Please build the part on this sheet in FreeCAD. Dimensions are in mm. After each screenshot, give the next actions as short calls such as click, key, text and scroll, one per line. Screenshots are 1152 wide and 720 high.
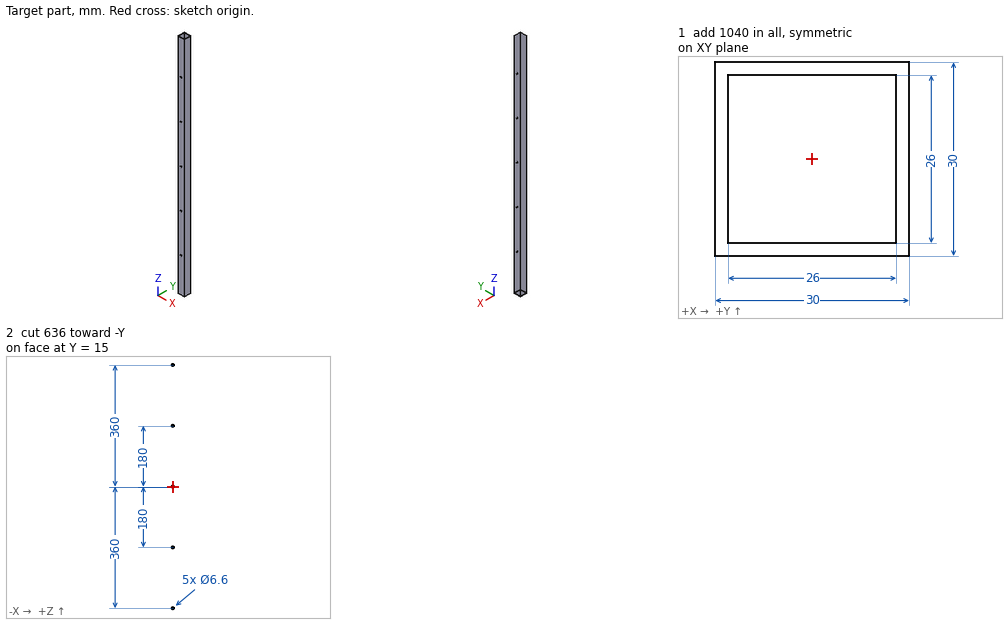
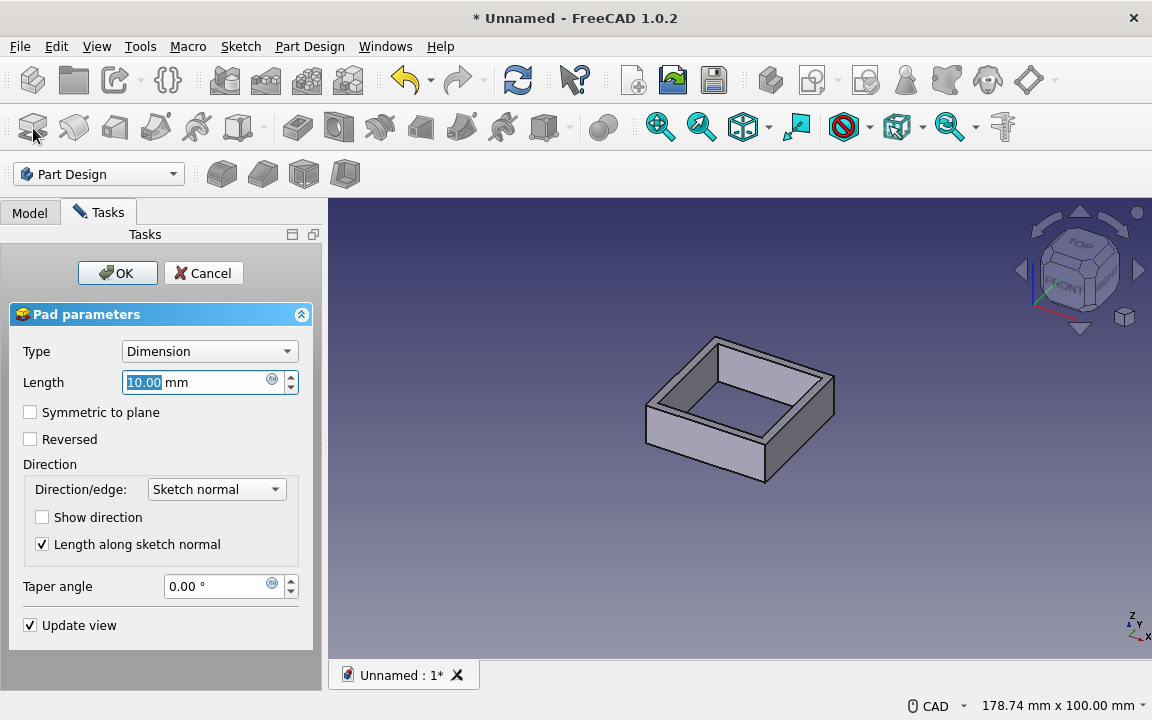
text(1040)
key(Tab)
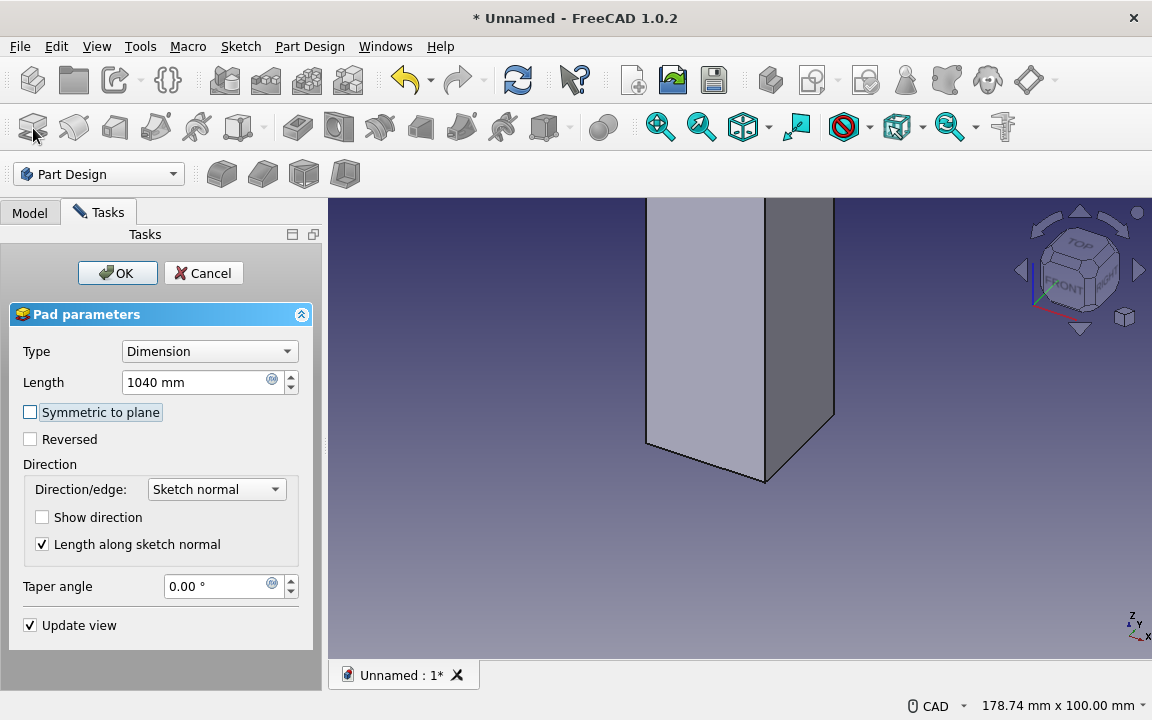
click(31, 412)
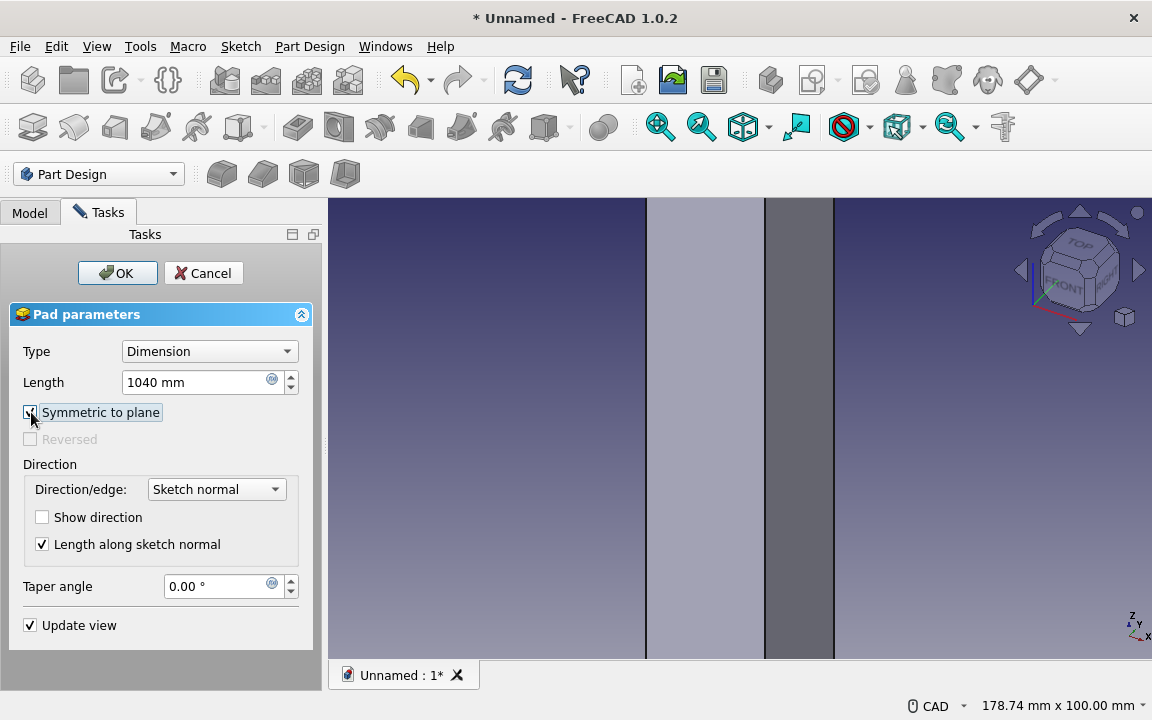
click(118, 273)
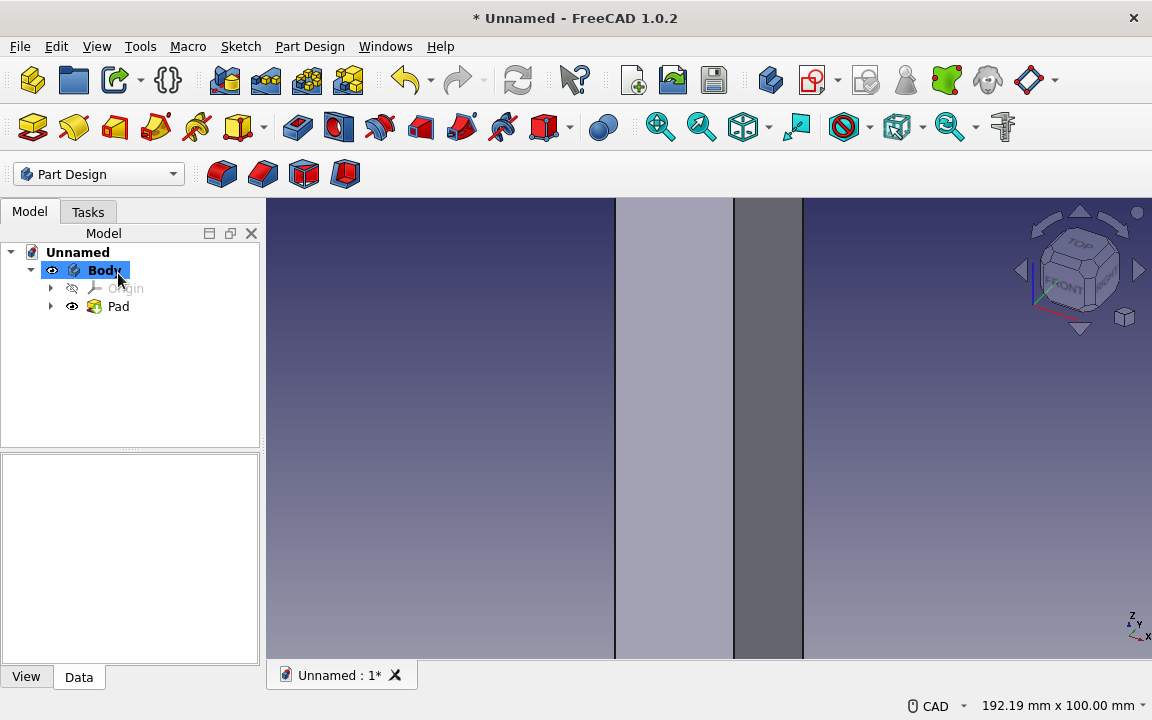
key(v)
key(f)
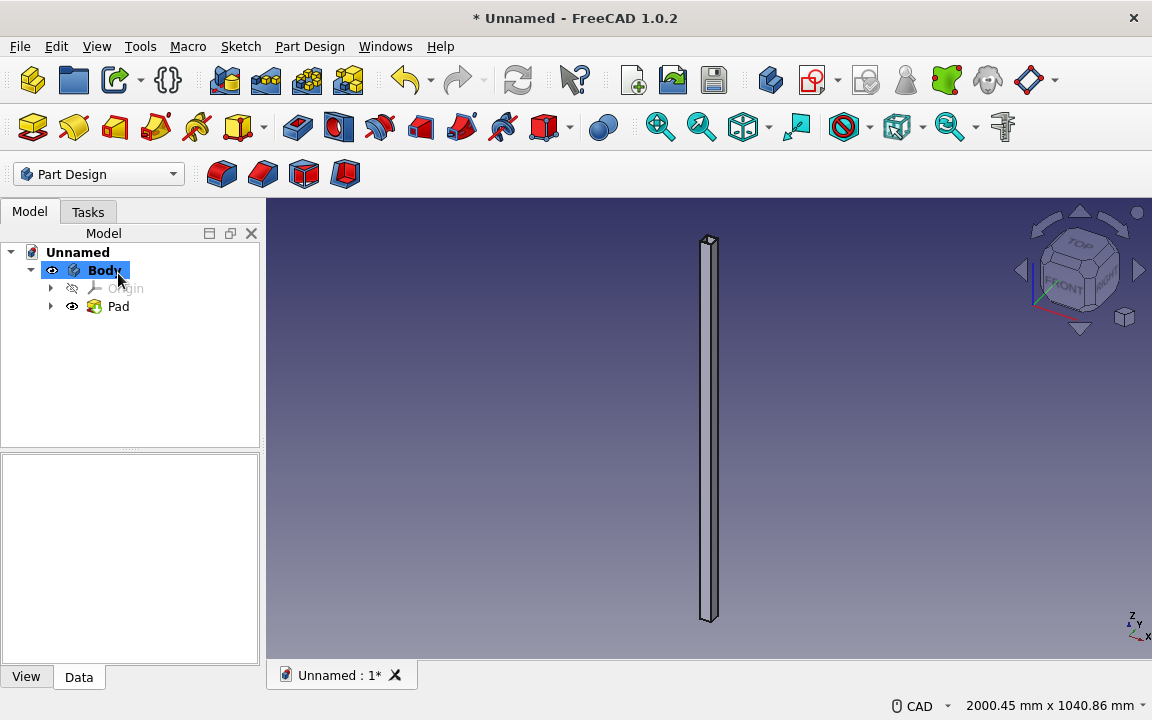
key(4)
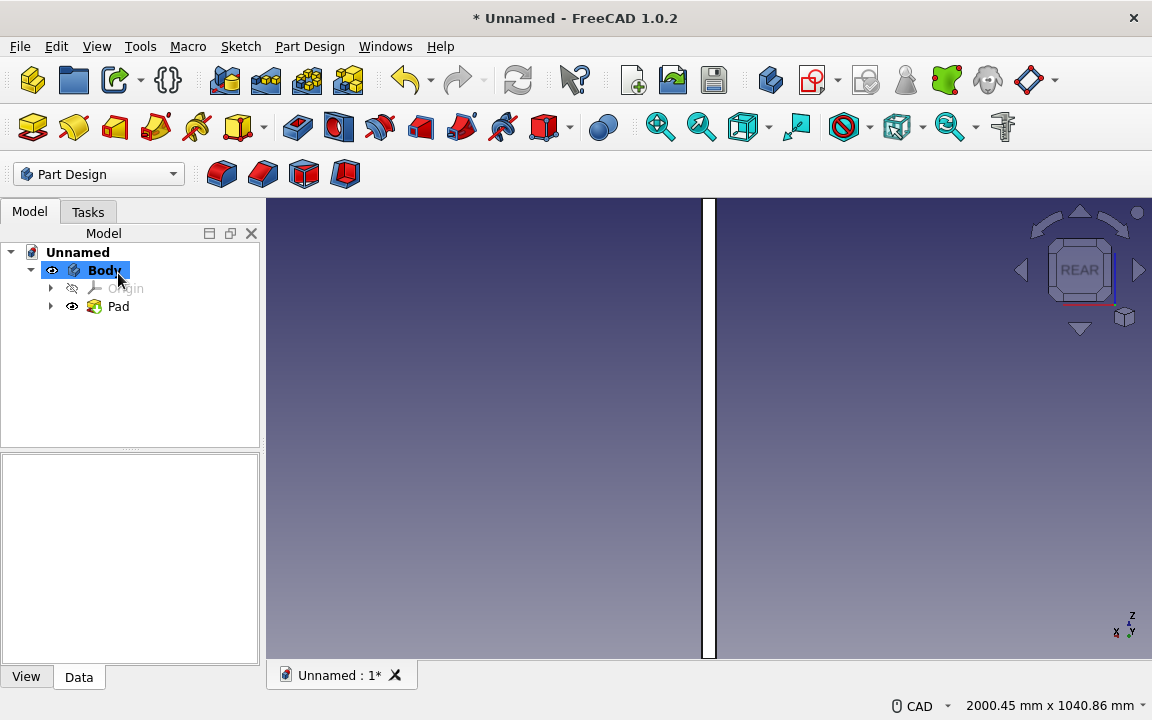
key(v)
key(f)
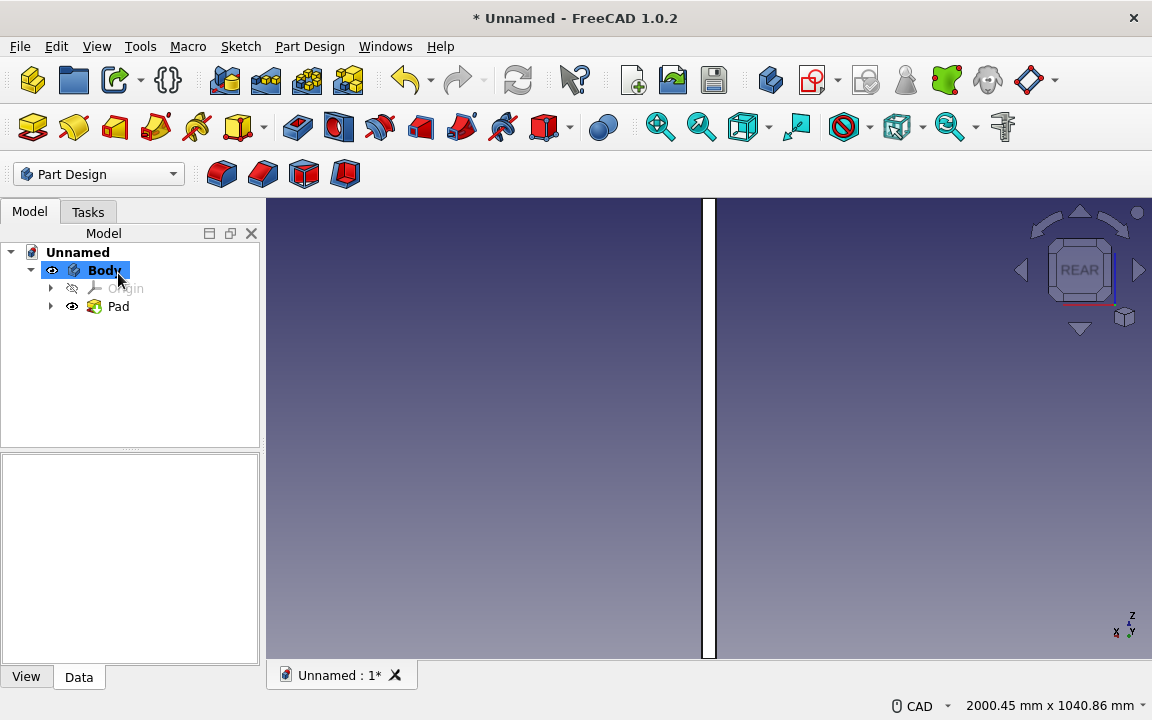
scroll(709, 230, up, 3)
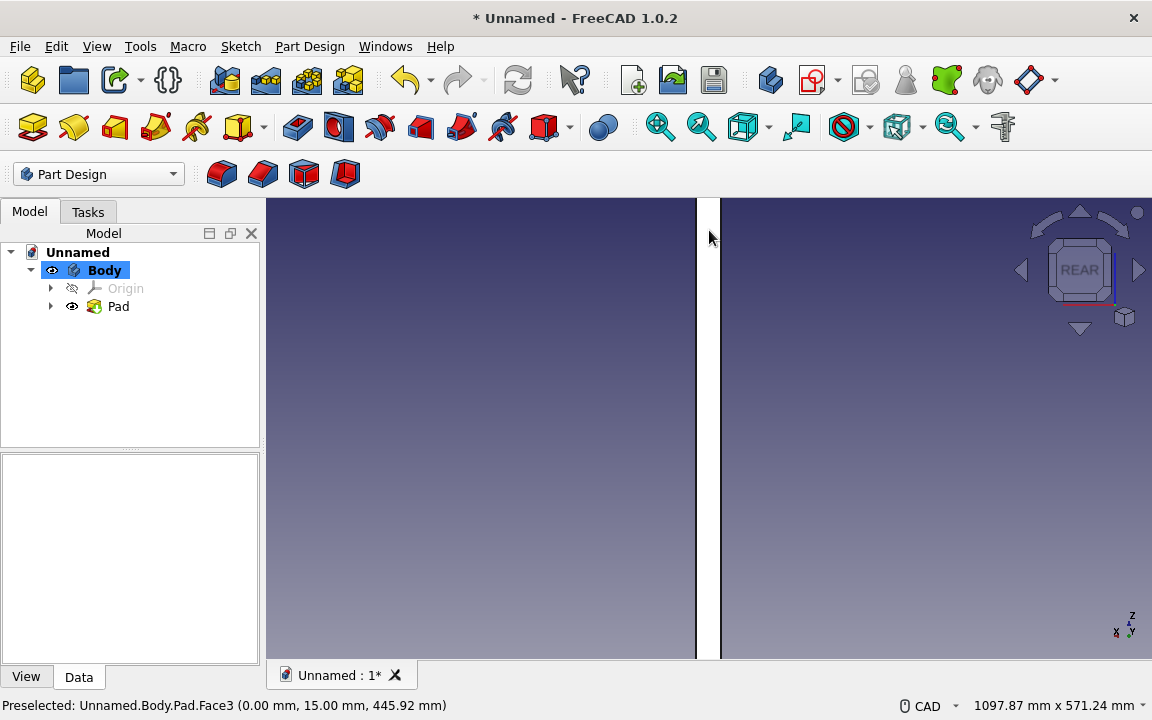
click(709, 231)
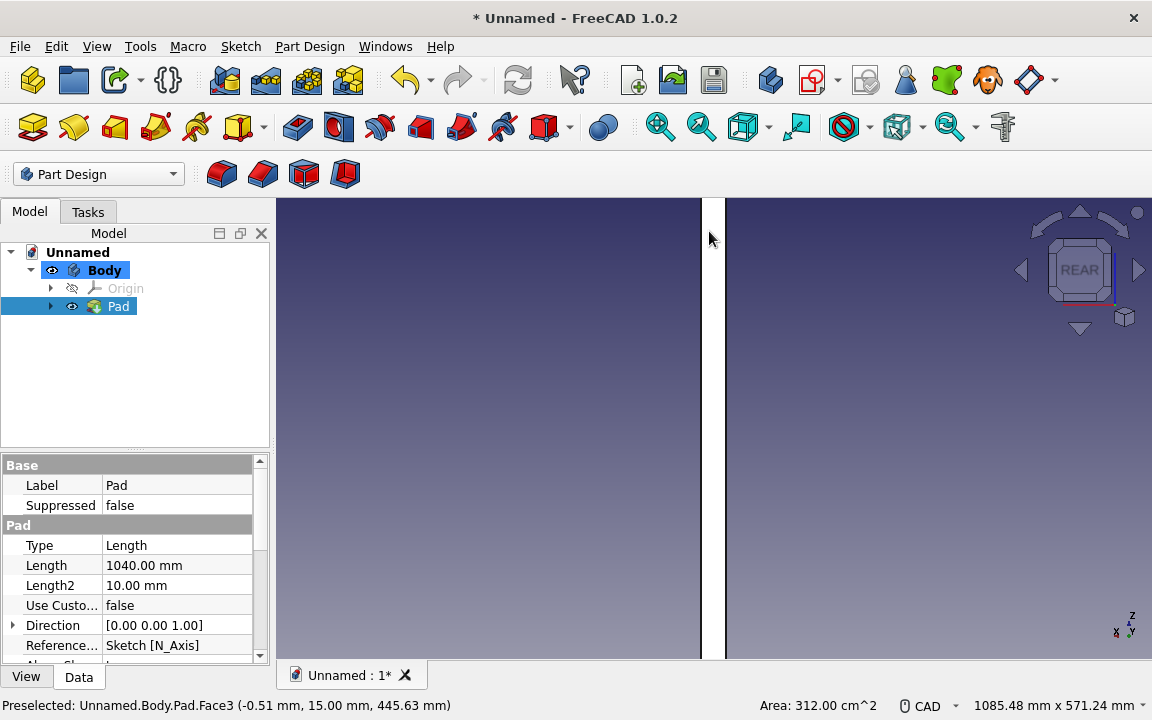
click(812, 80)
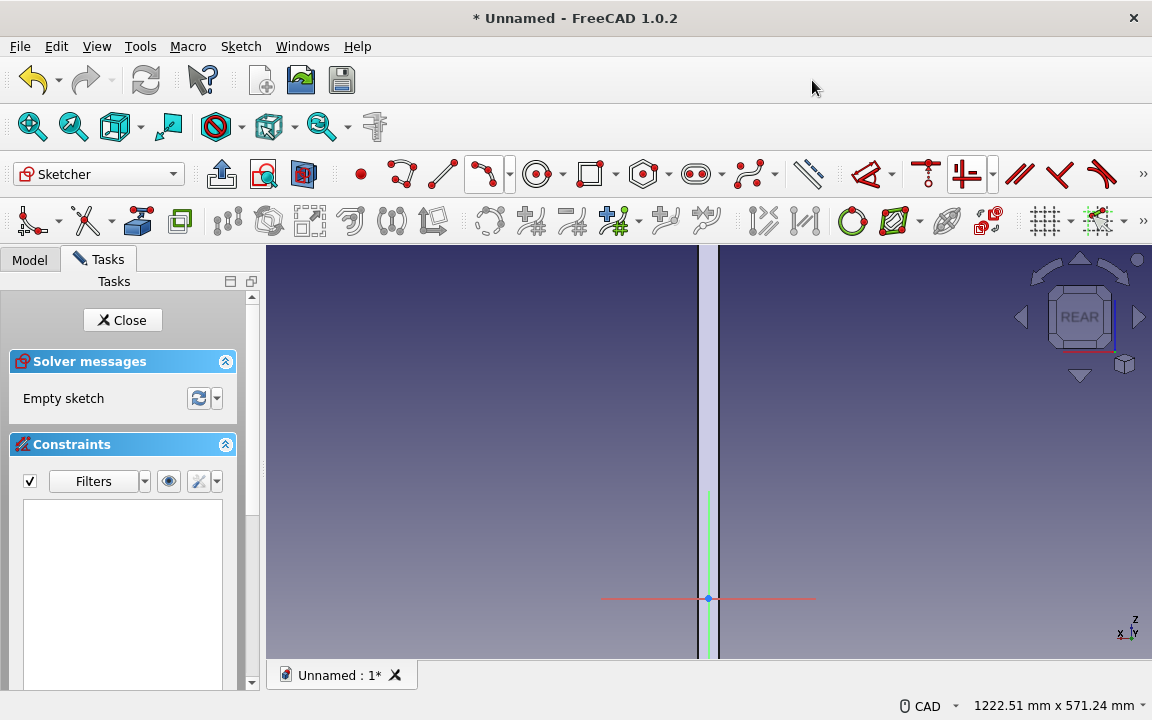
scroll(585, 332, down, 4)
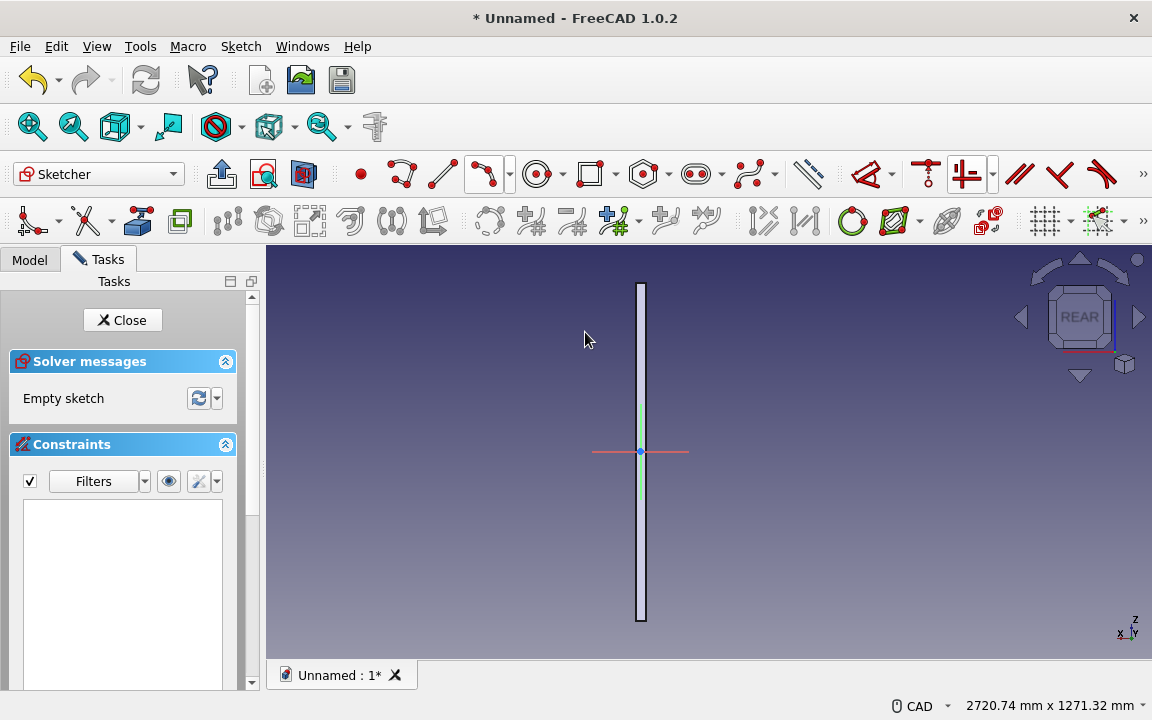
click(536, 174)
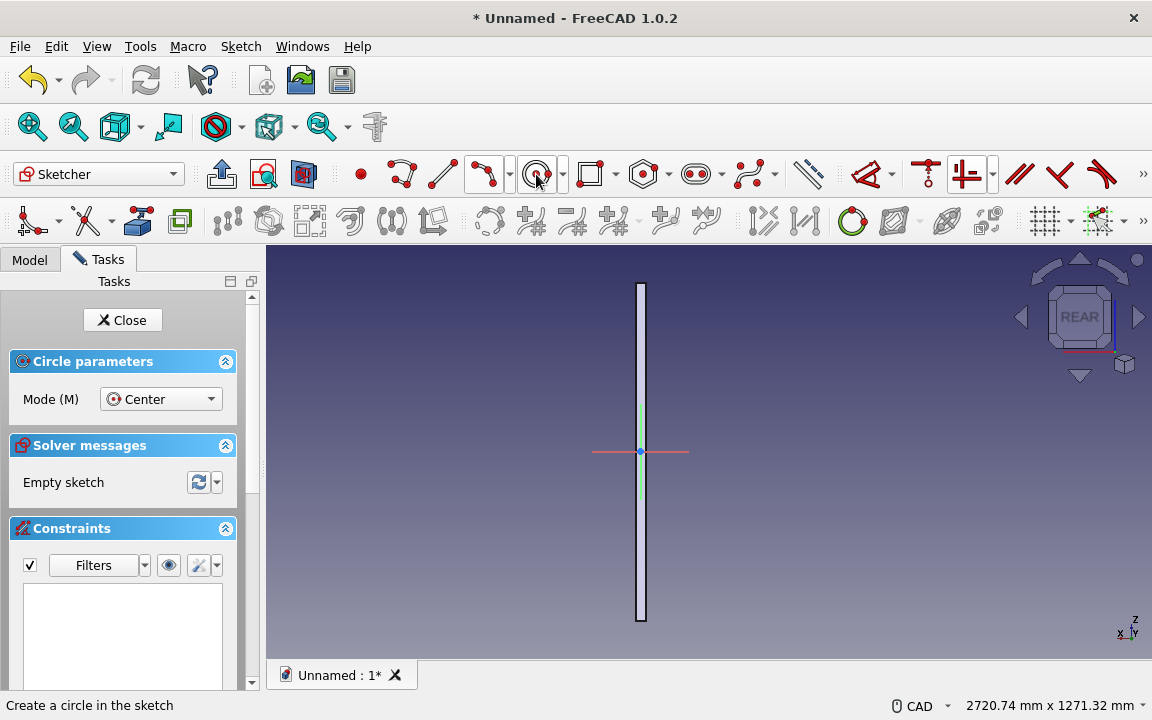
scroll(641, 569, up, 16)